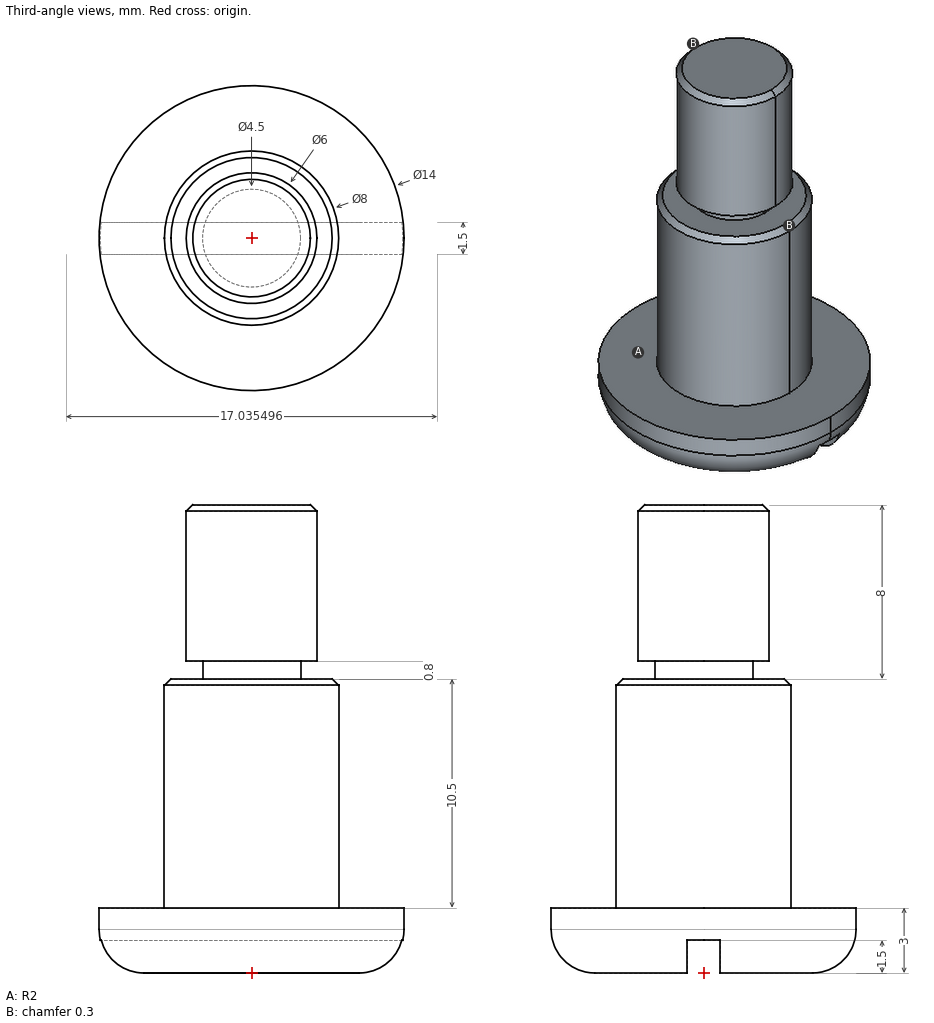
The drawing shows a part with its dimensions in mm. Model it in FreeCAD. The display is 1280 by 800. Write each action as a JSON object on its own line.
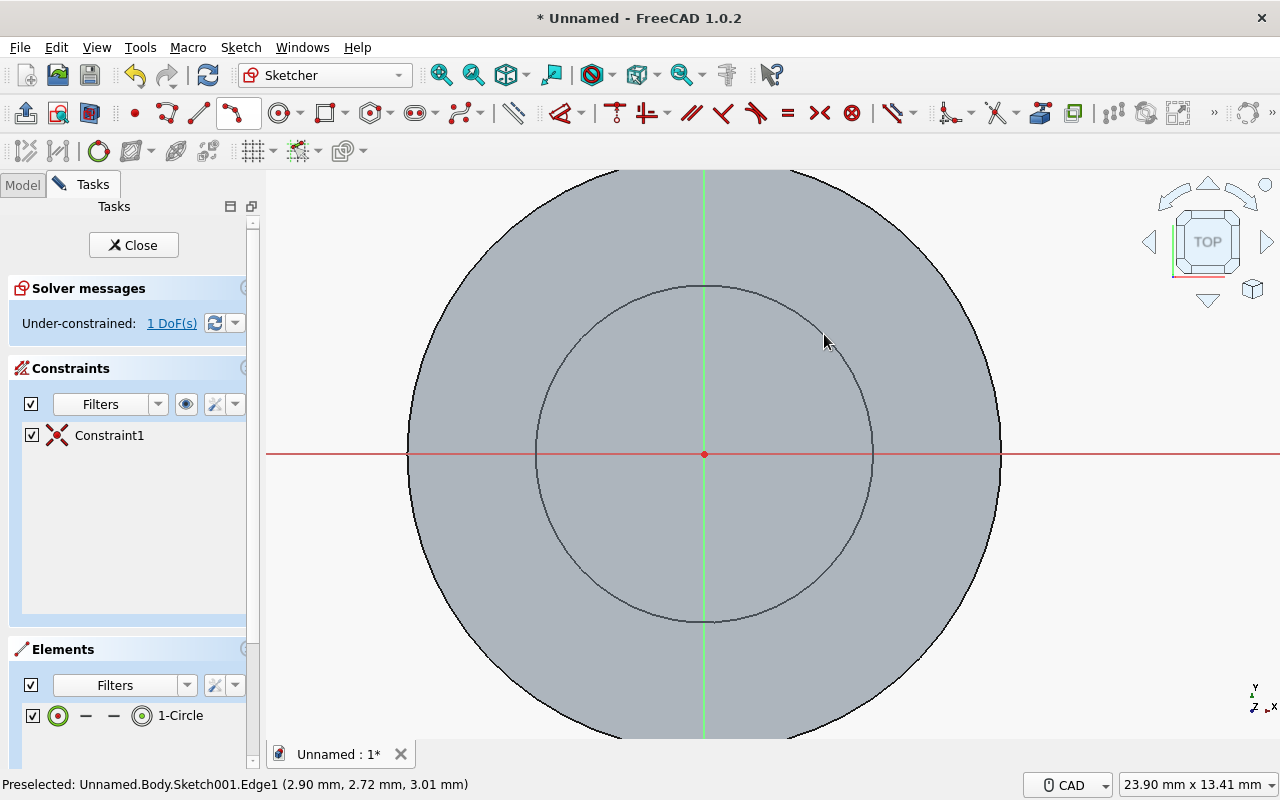
{"action": "left_click", "coordinate": [560, 114]}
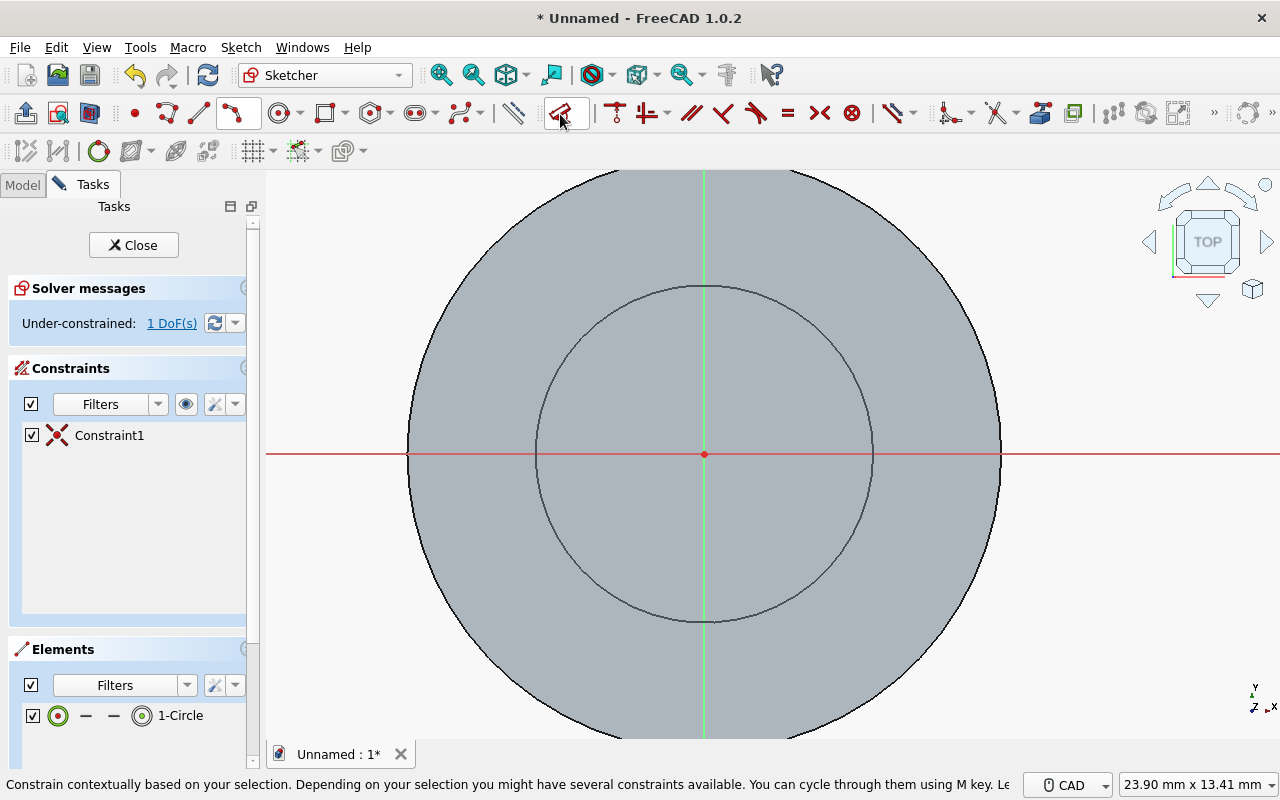
{"action": "left_click", "coordinate": [823, 334]}
{"action": "left_click", "coordinate": [846, 311]}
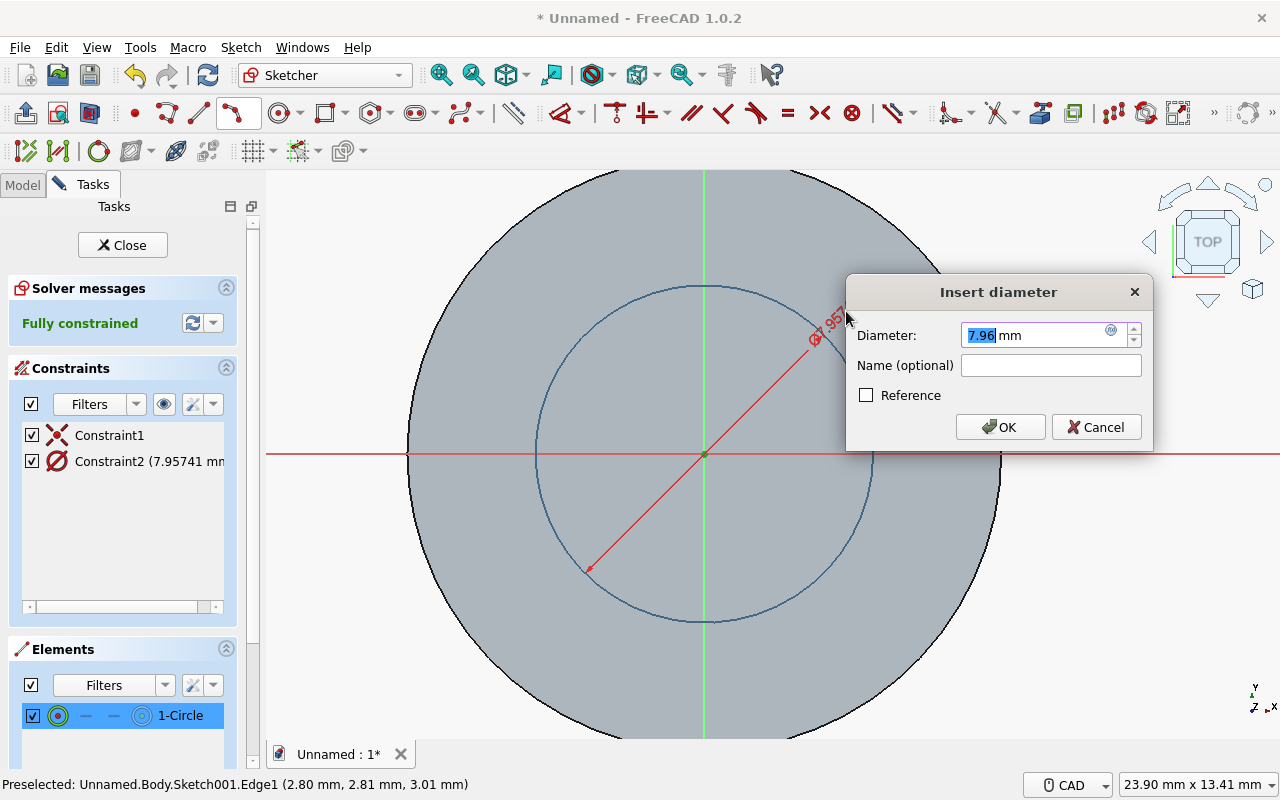
{"action": "type", "text": "8"}
{"action": "key", "text": "Return"}
{"action": "key", "text": "Escape"}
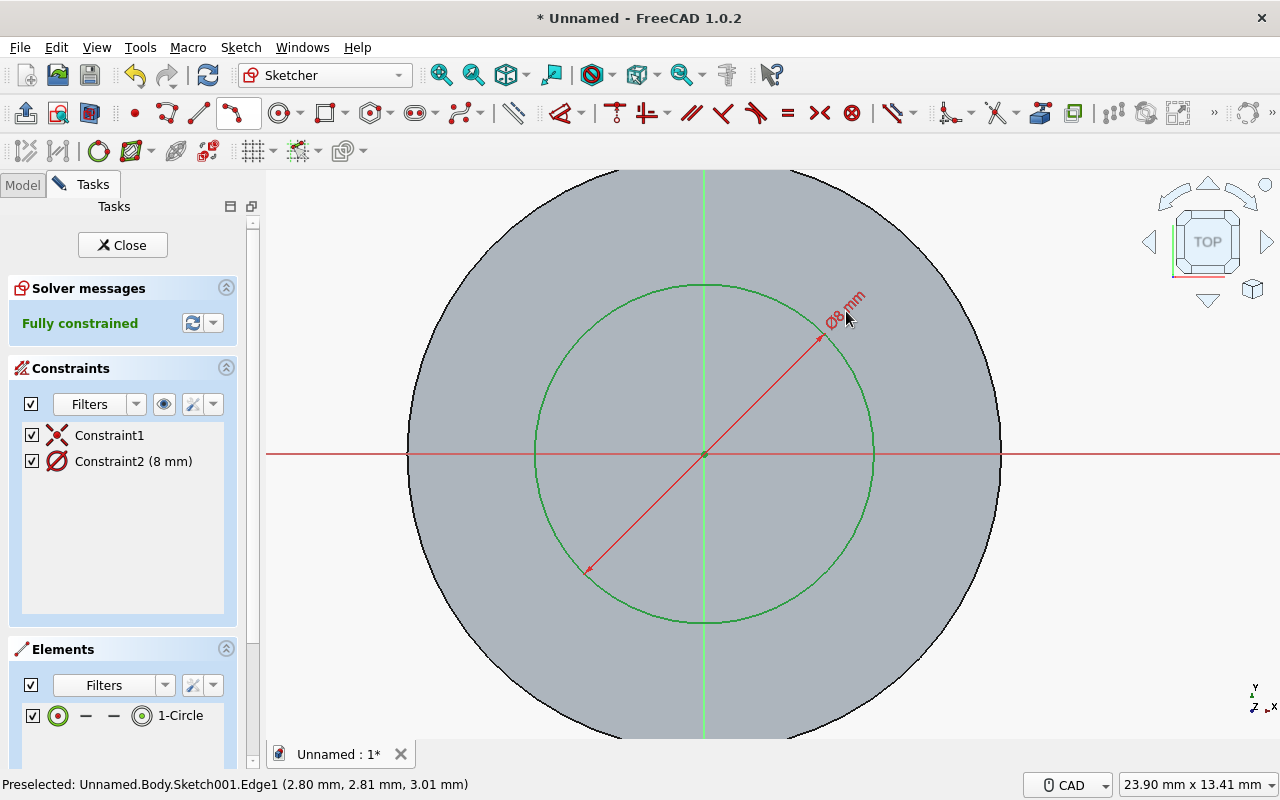
{"action": "left_click", "coordinate": [123, 245]}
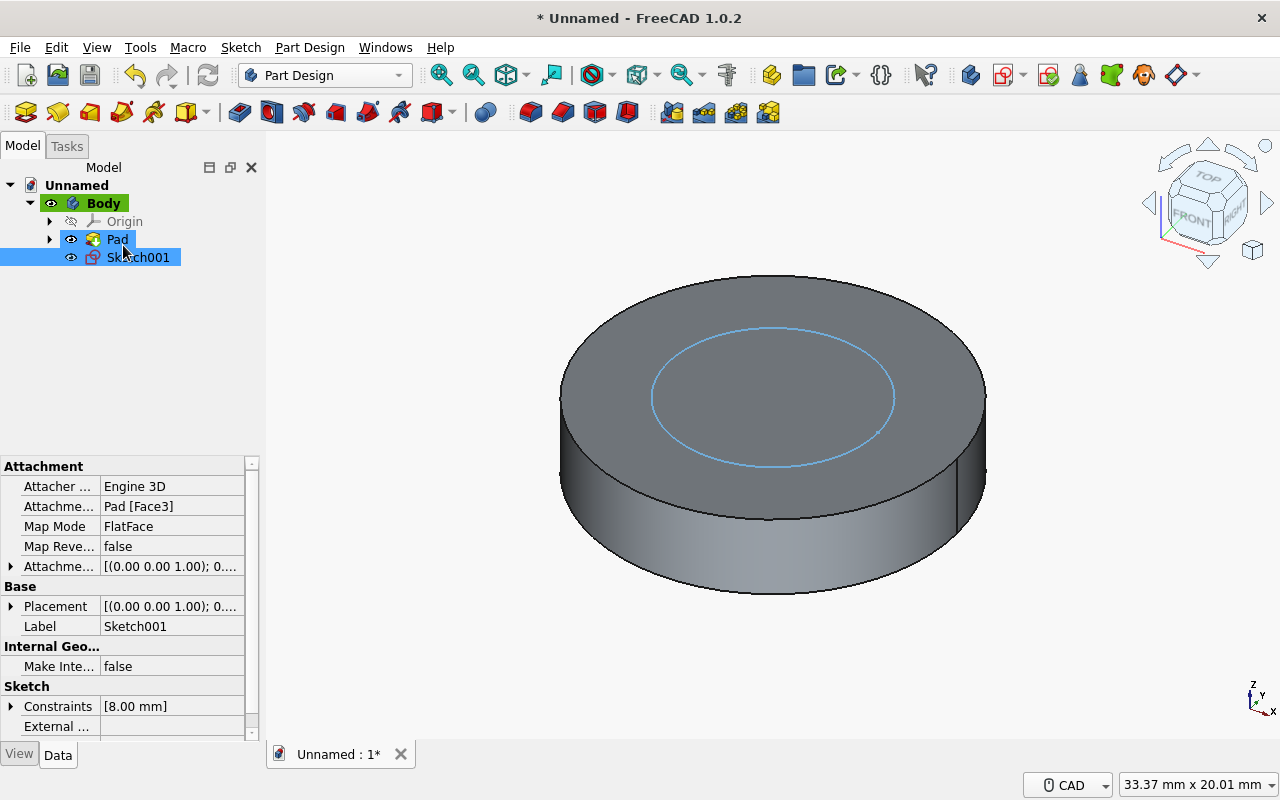
{"action": "left_click", "coordinate": [26, 112]}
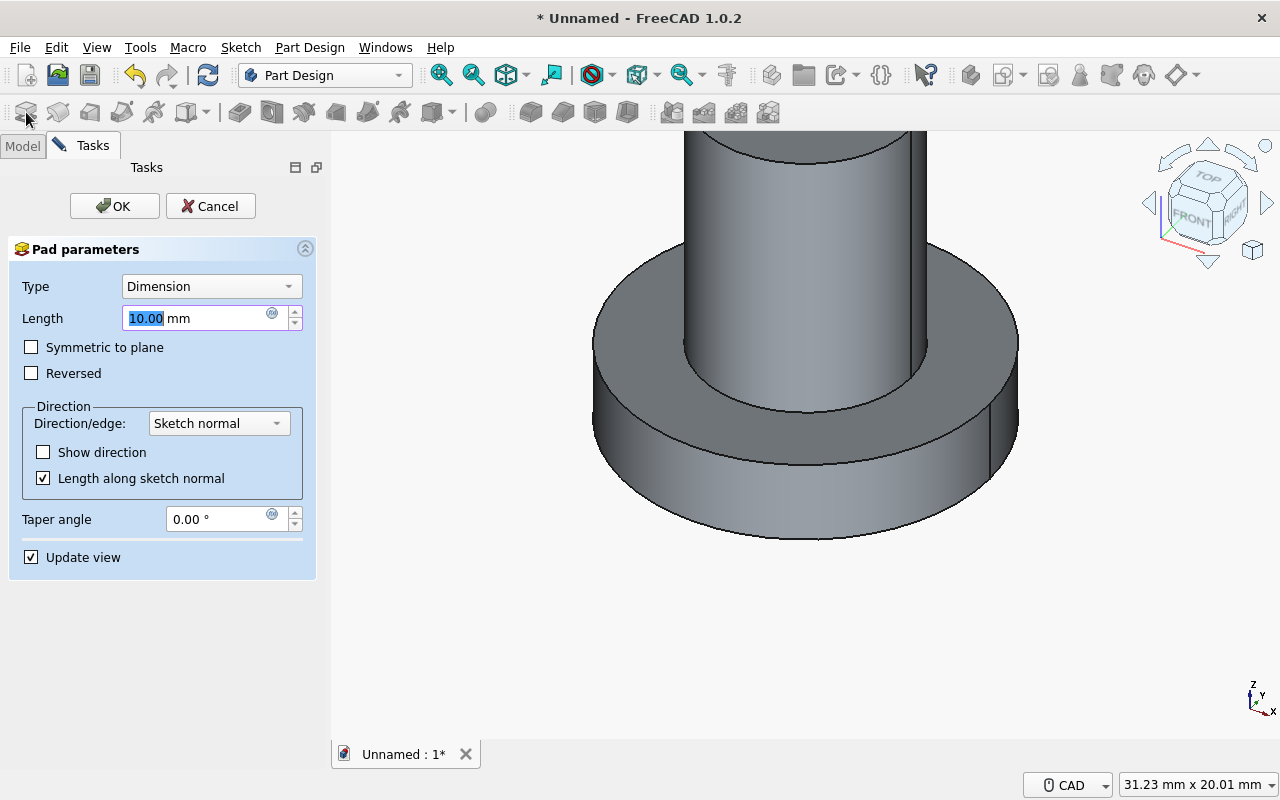
{"action": "type", "text": "10.5"}
{"action": "key", "text": "Tab"}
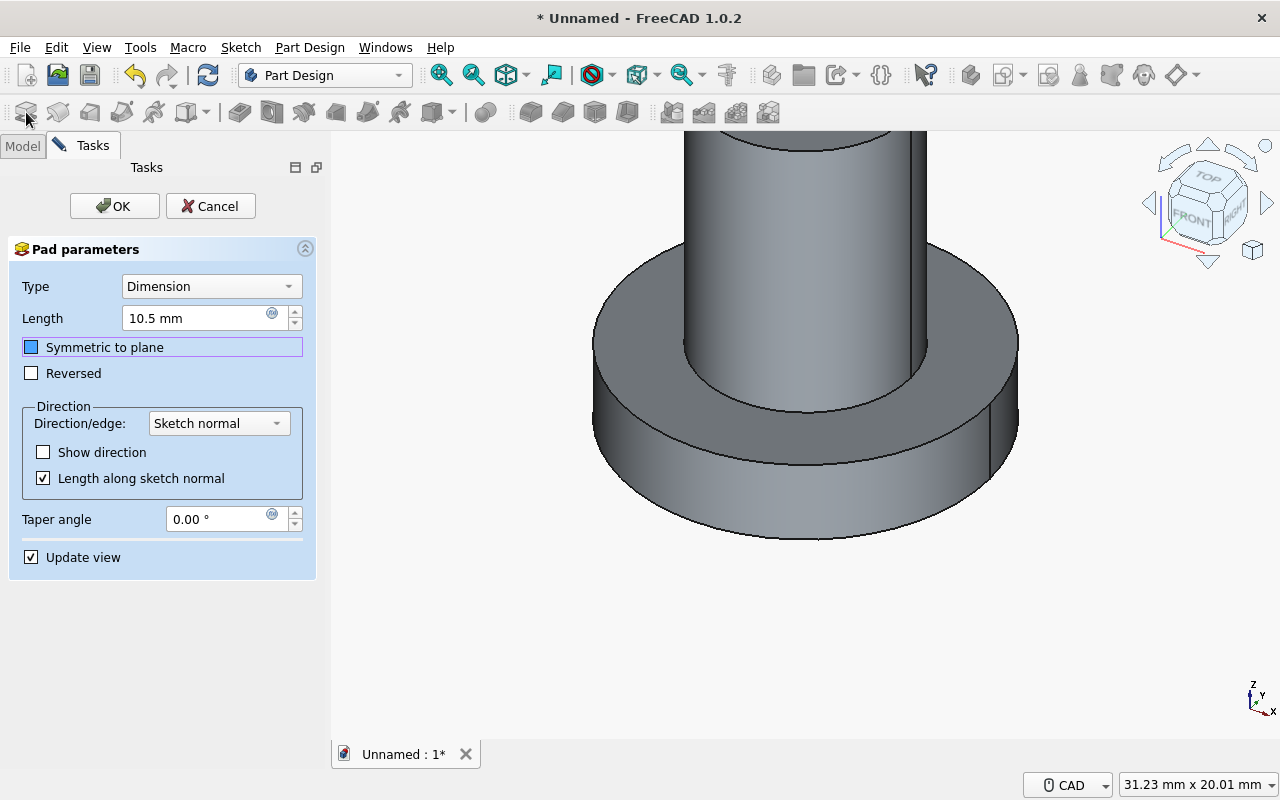
{"action": "left_click", "coordinate": [115, 206]}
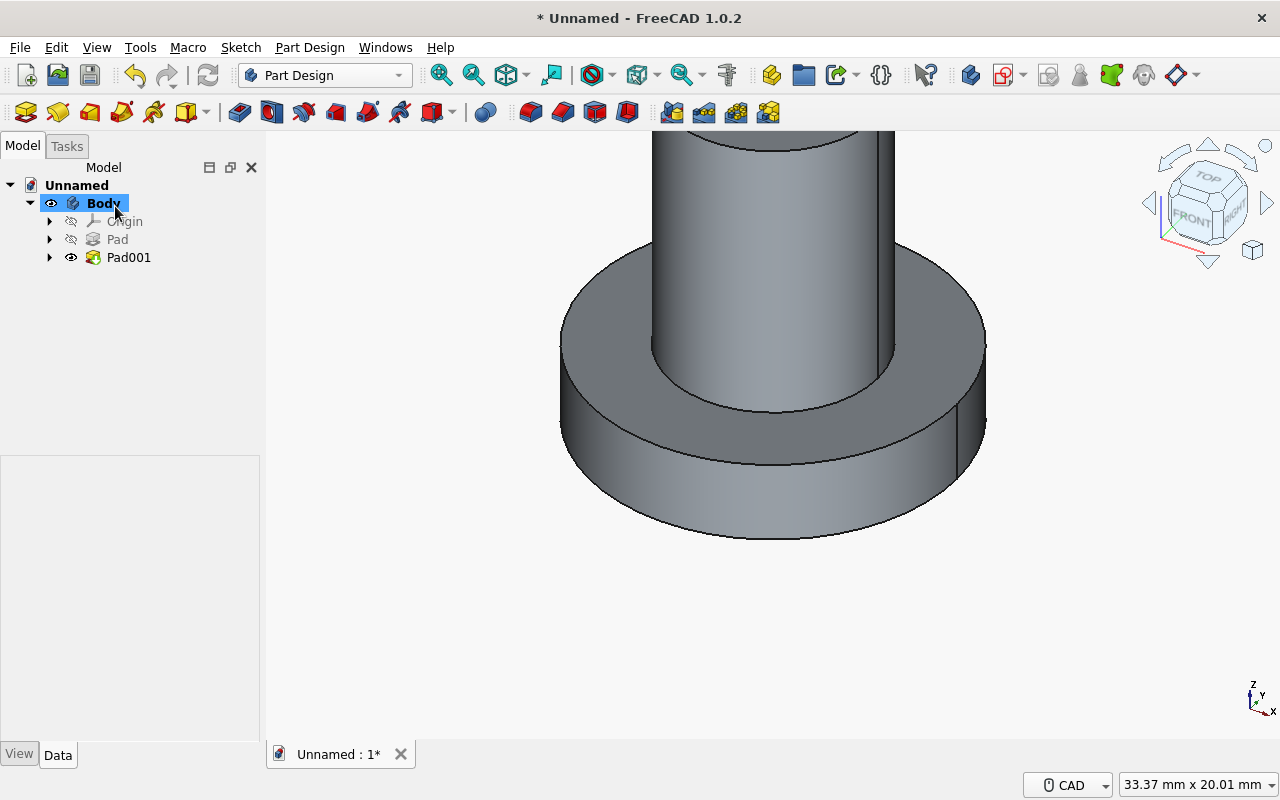
{"action": "left_click", "coordinate": [442, 76]}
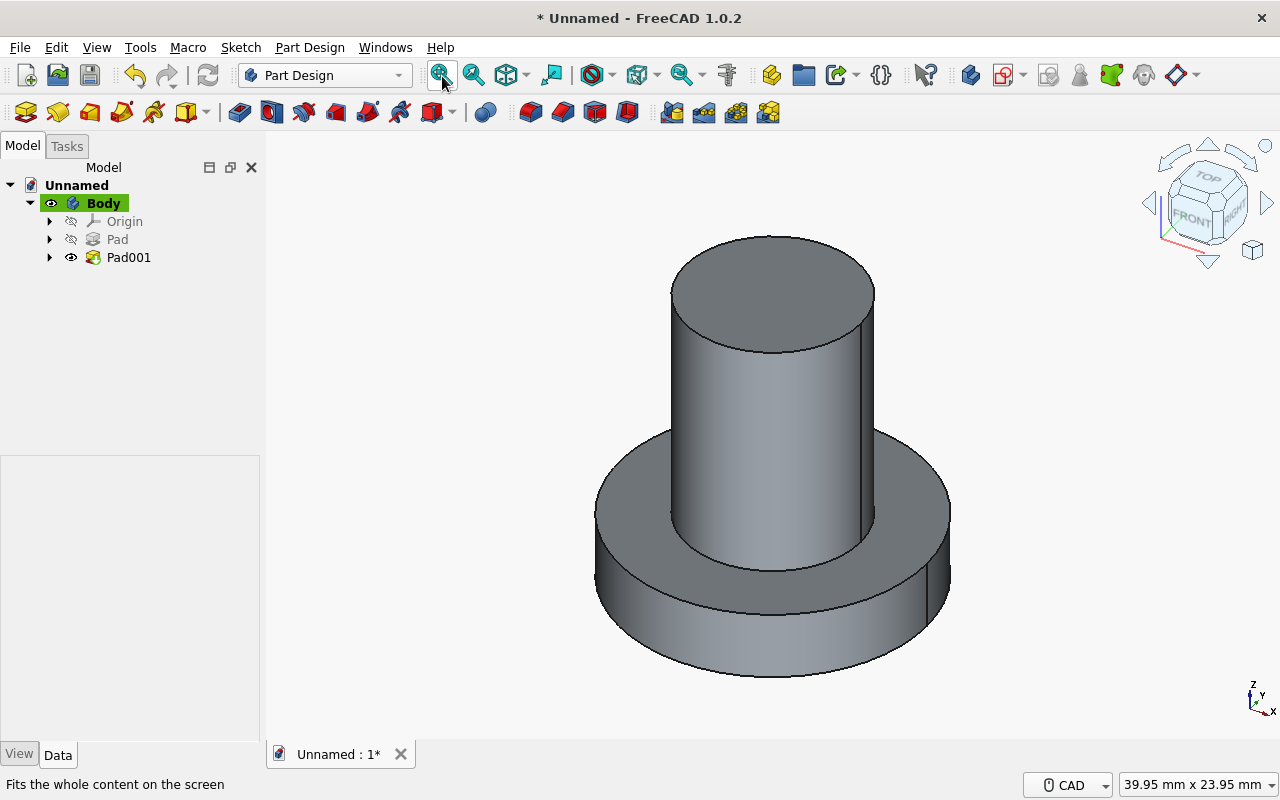
{"action": "left_click", "coordinate": [773, 294]}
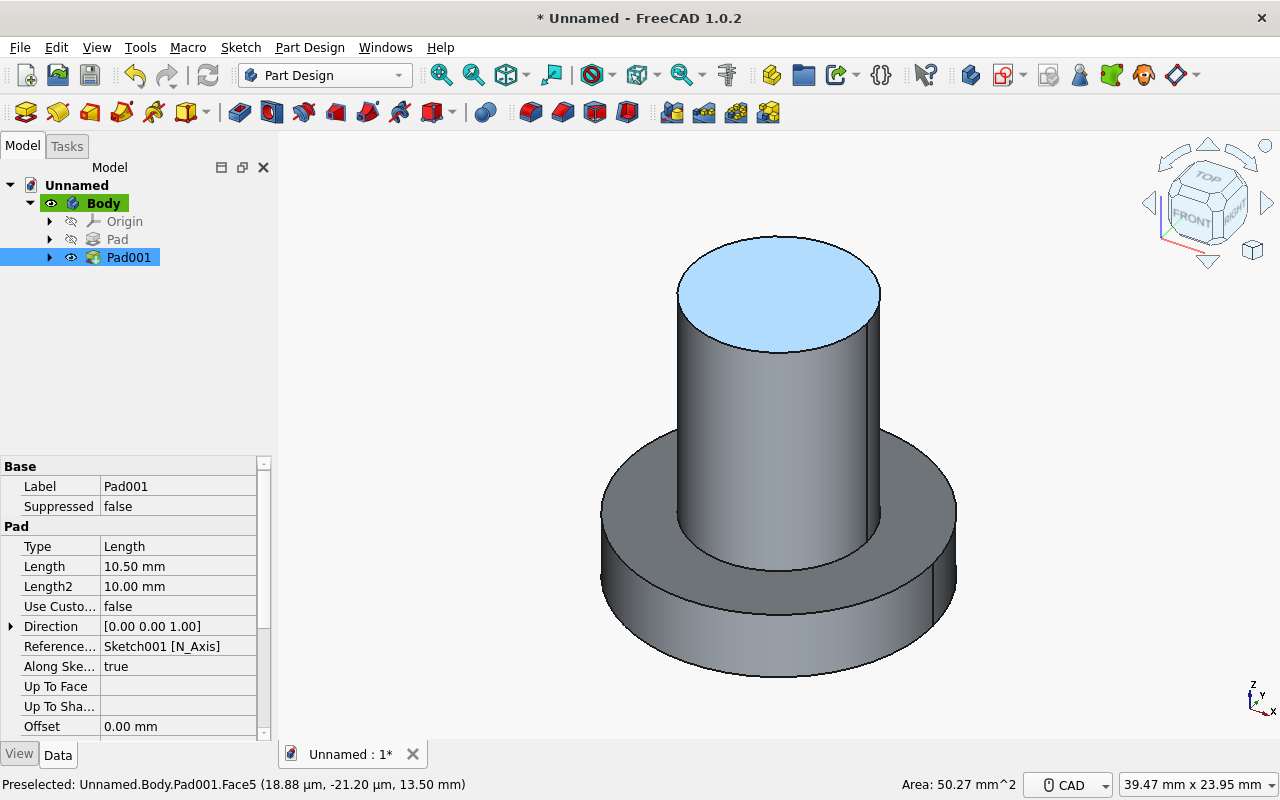
{"action": "left_click", "coordinate": [1004, 76]}